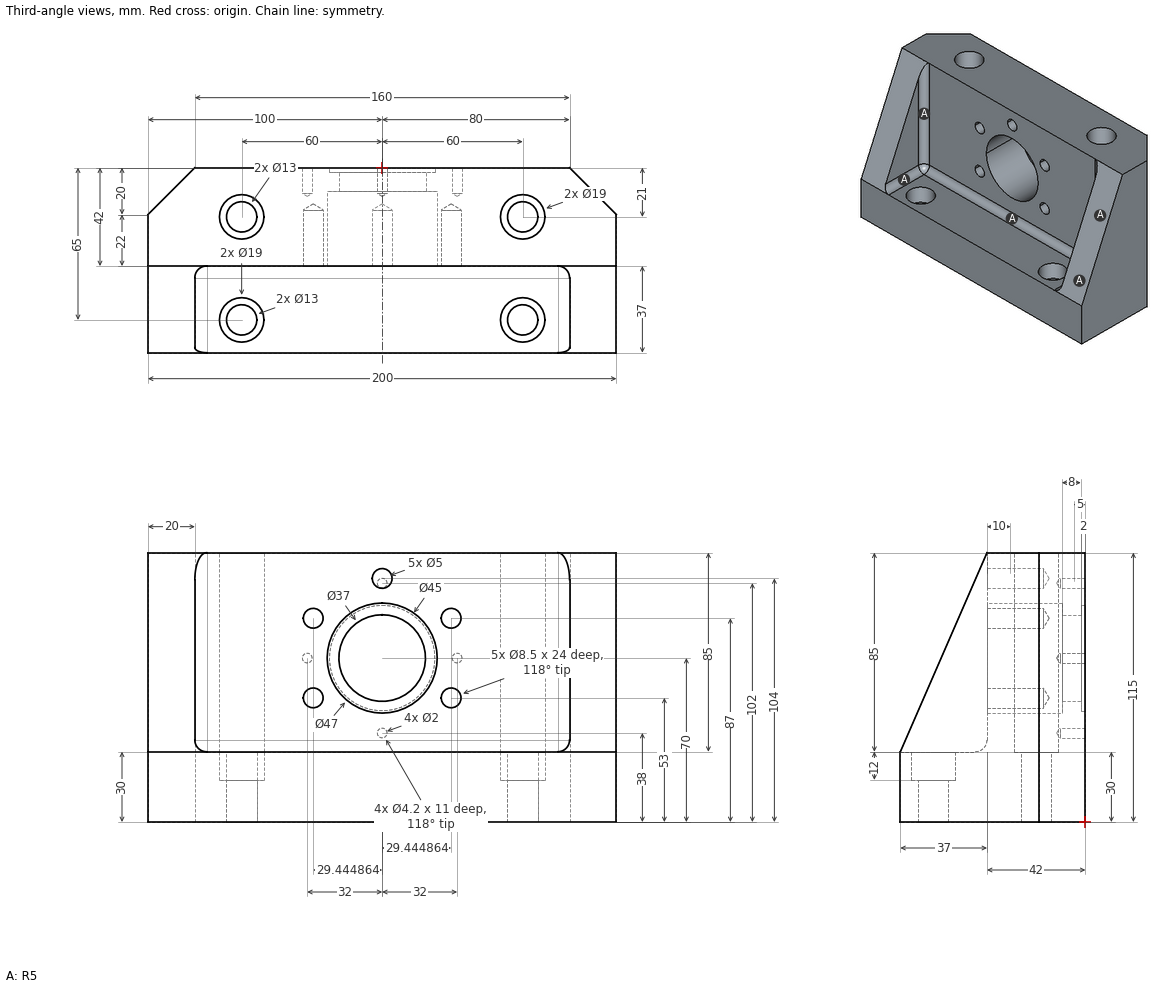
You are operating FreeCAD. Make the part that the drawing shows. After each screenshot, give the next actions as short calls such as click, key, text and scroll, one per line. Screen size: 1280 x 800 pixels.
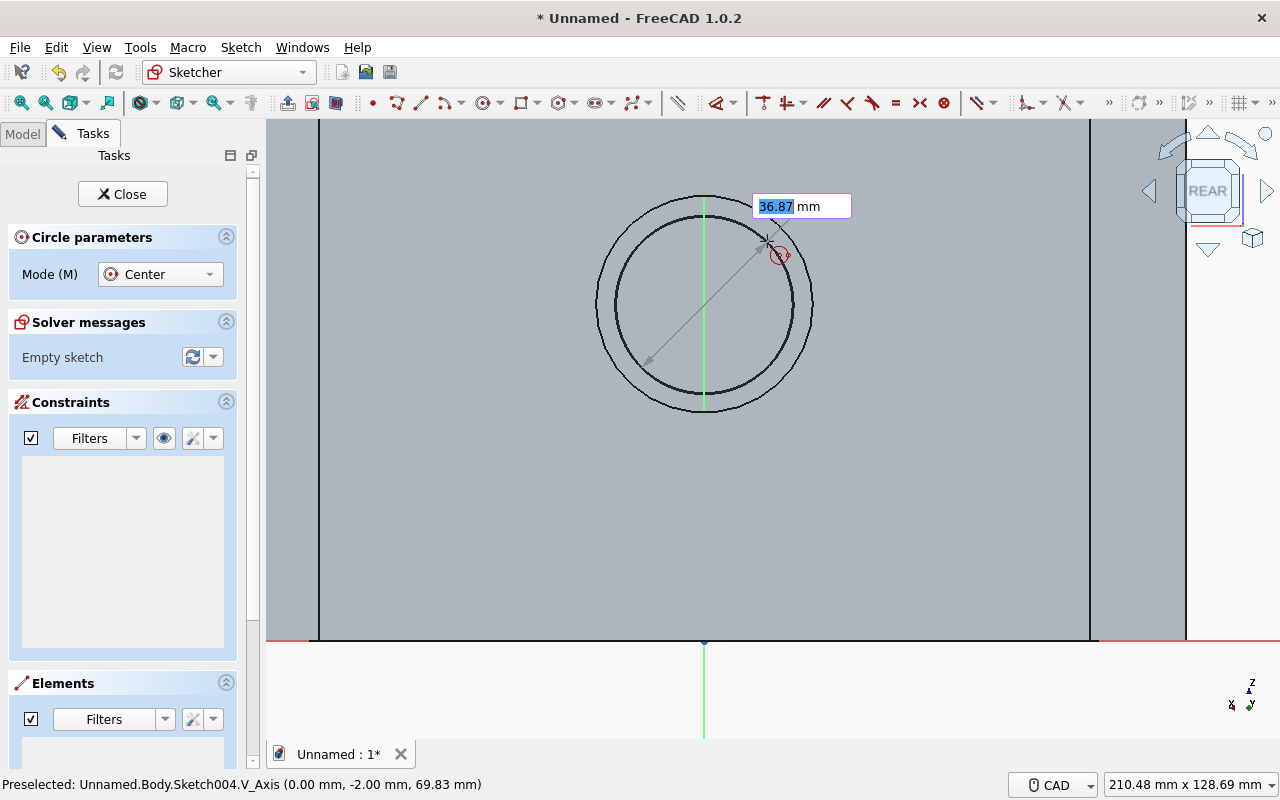
text(37)
key(Return)
key(Escape)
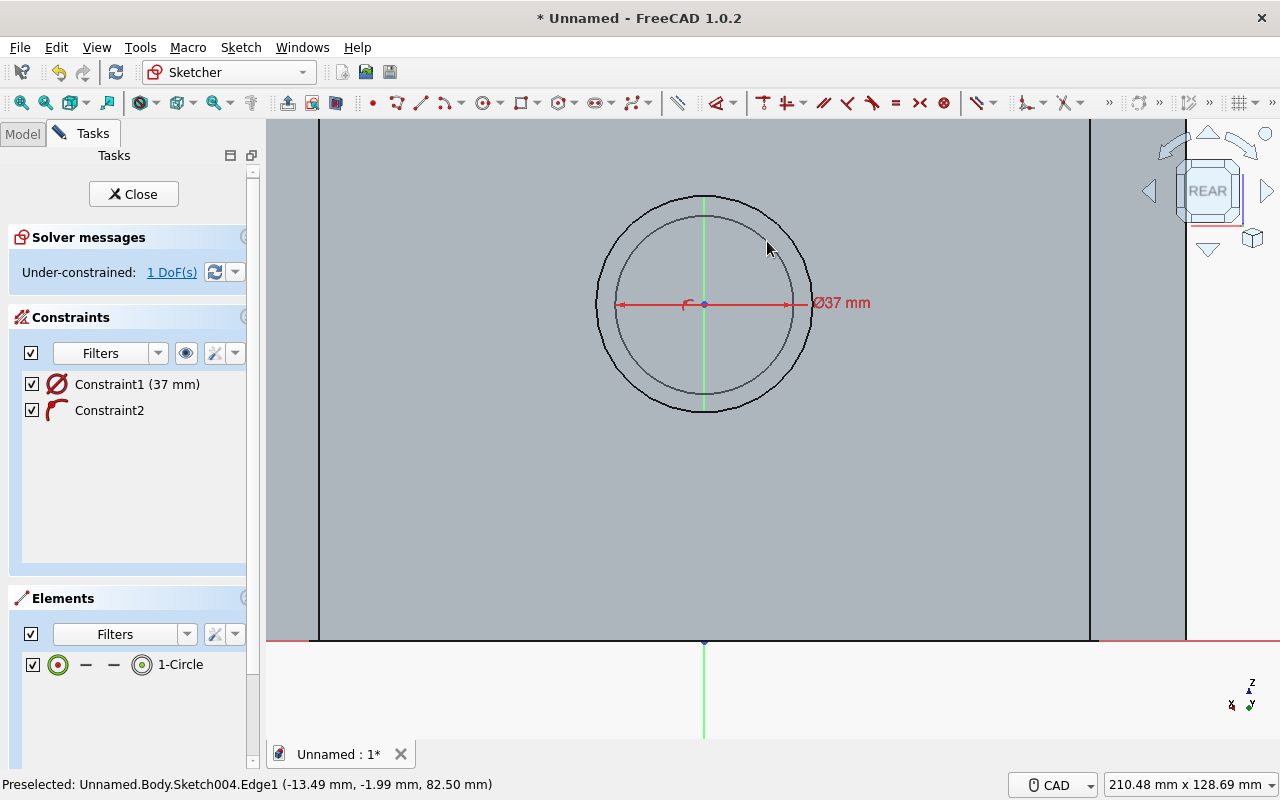
click(716, 104)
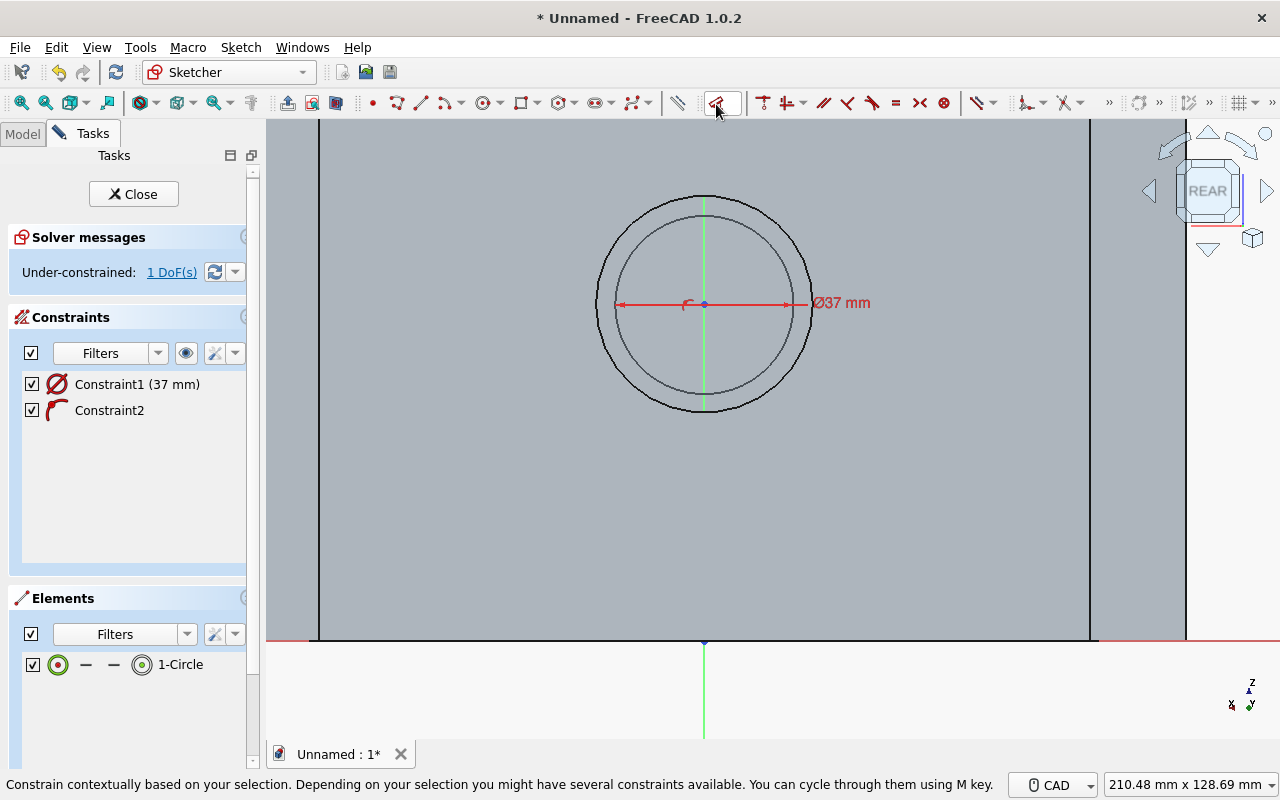
click(704, 305)
click(738, 473)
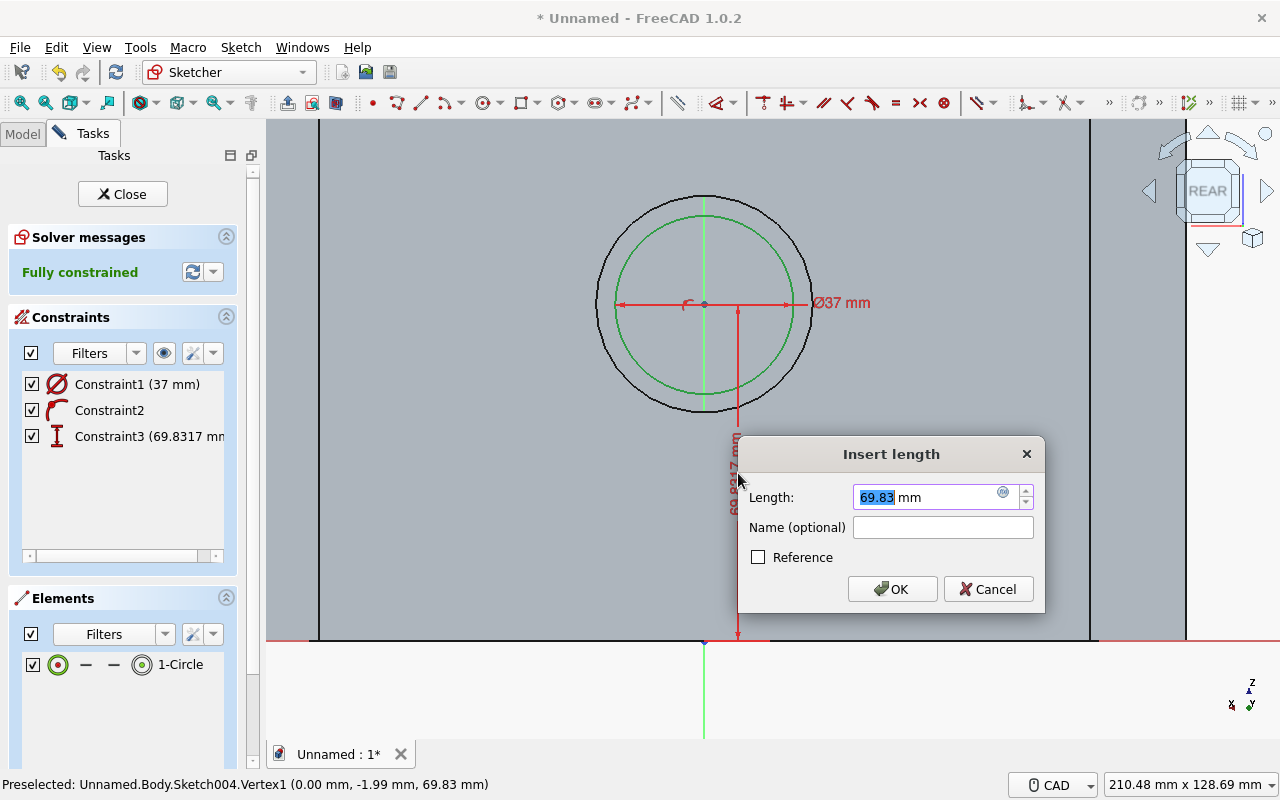
text(70)
key(Return)
key(Escape)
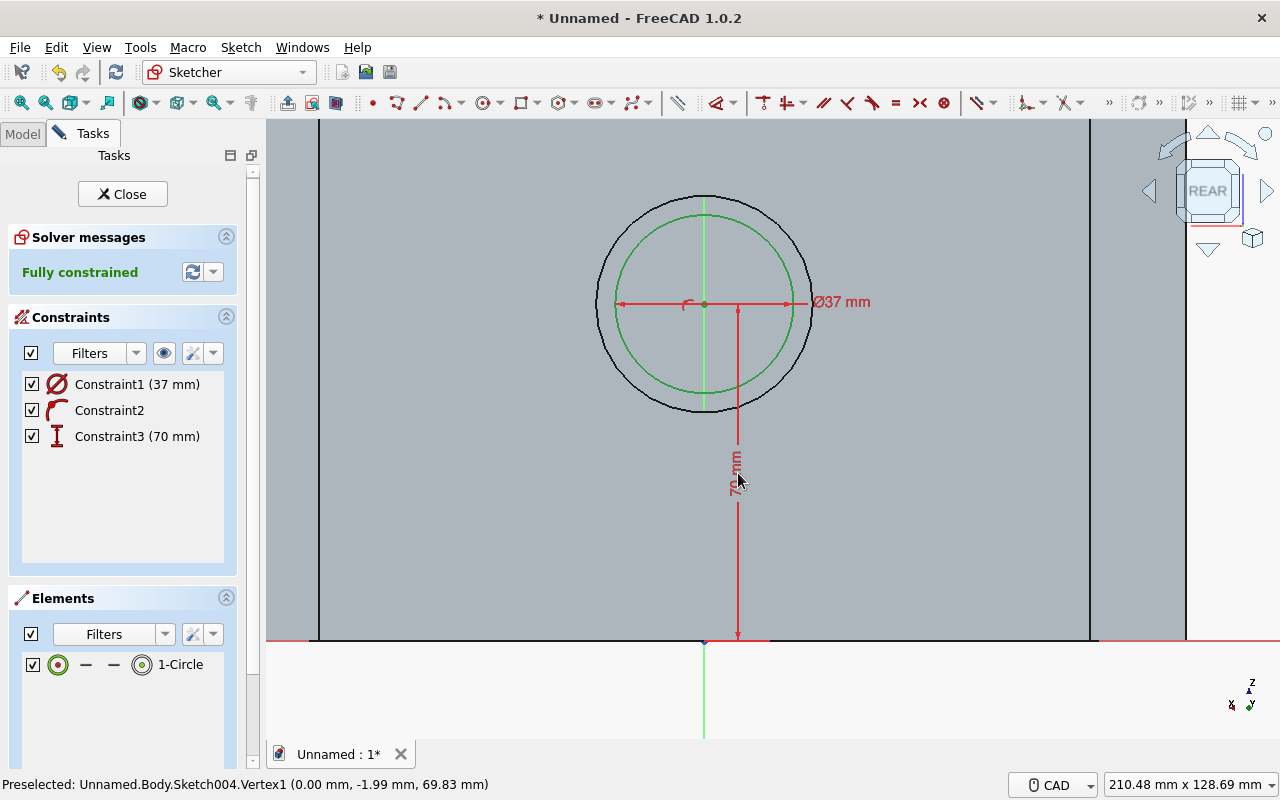
click(123, 194)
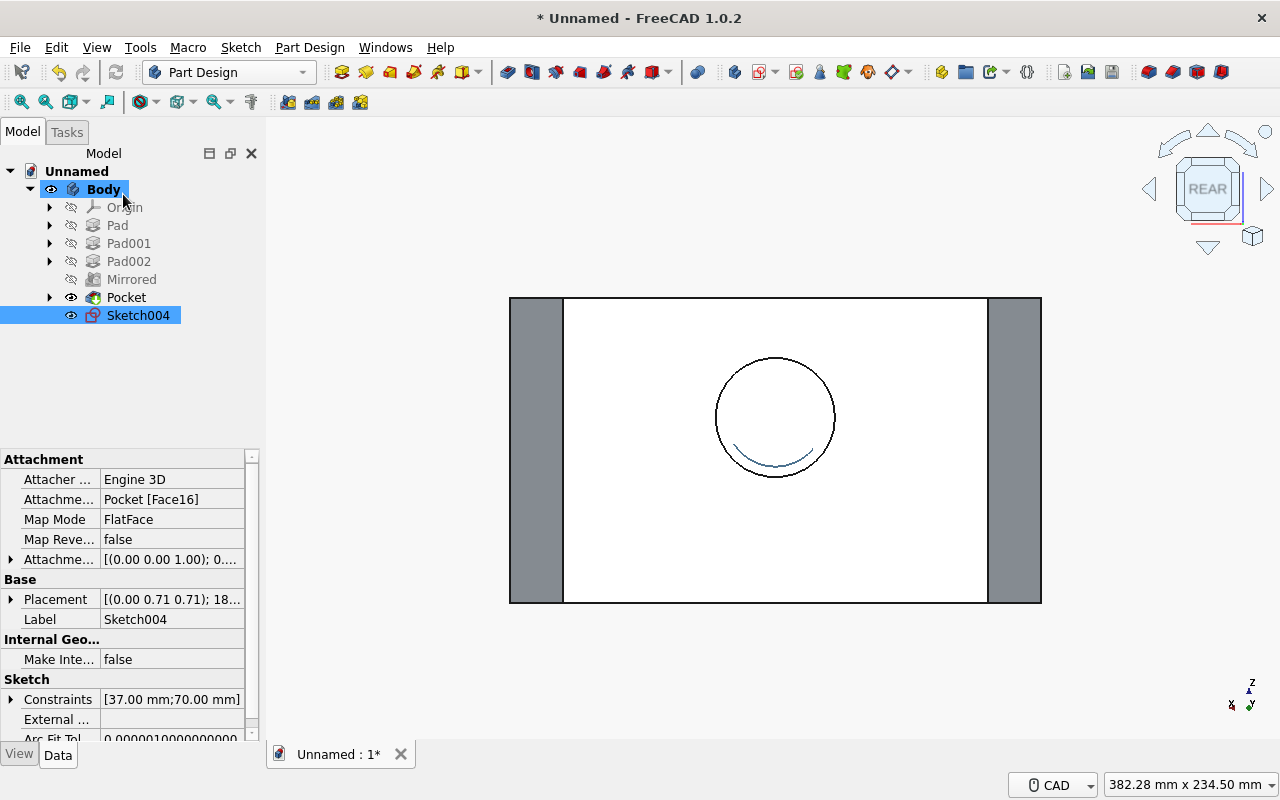
click(508, 72)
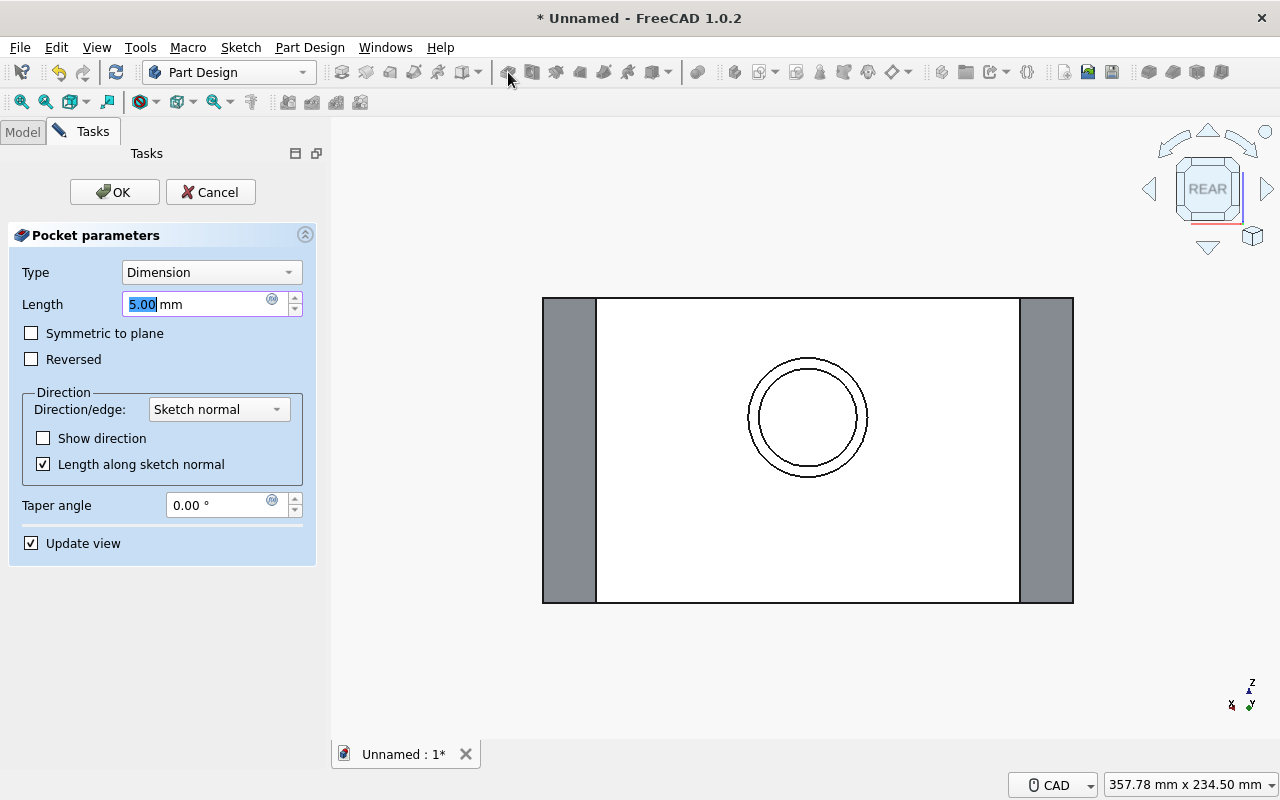
text(8)
key(Tab)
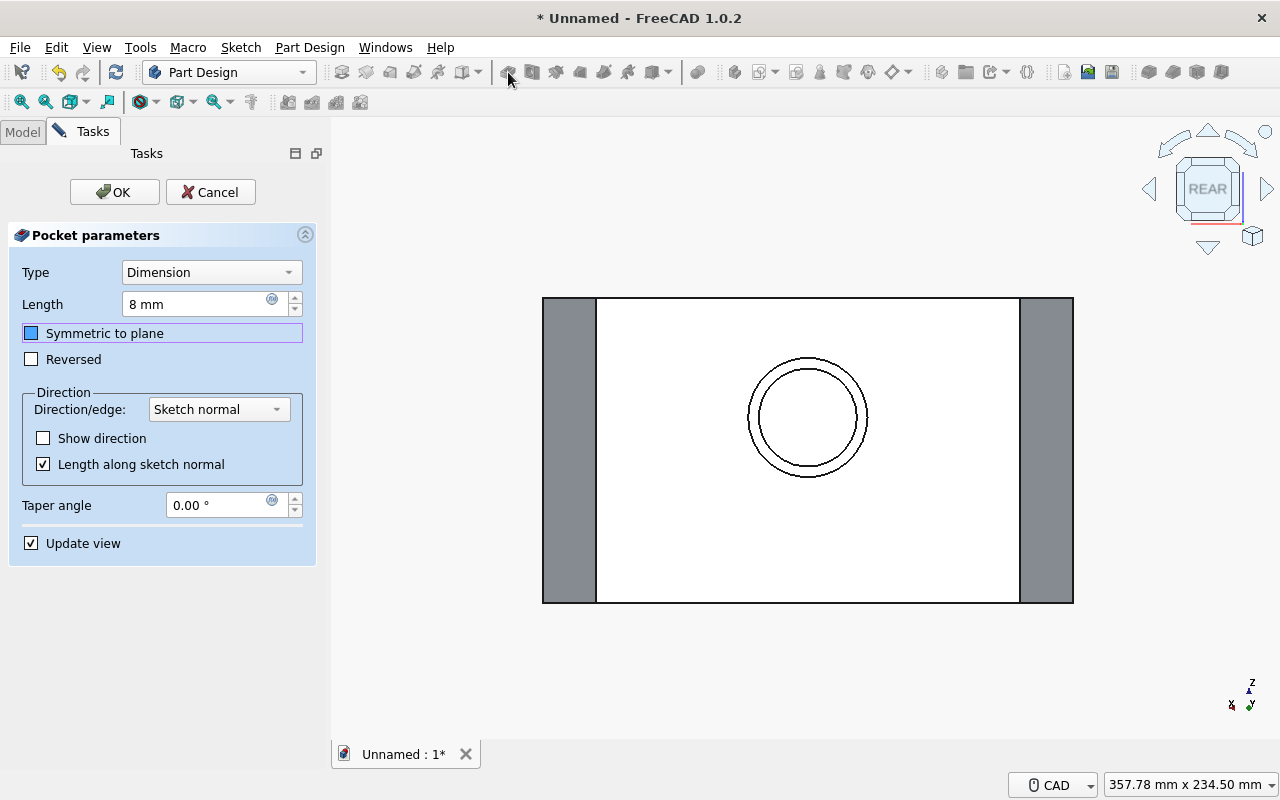
click(115, 192)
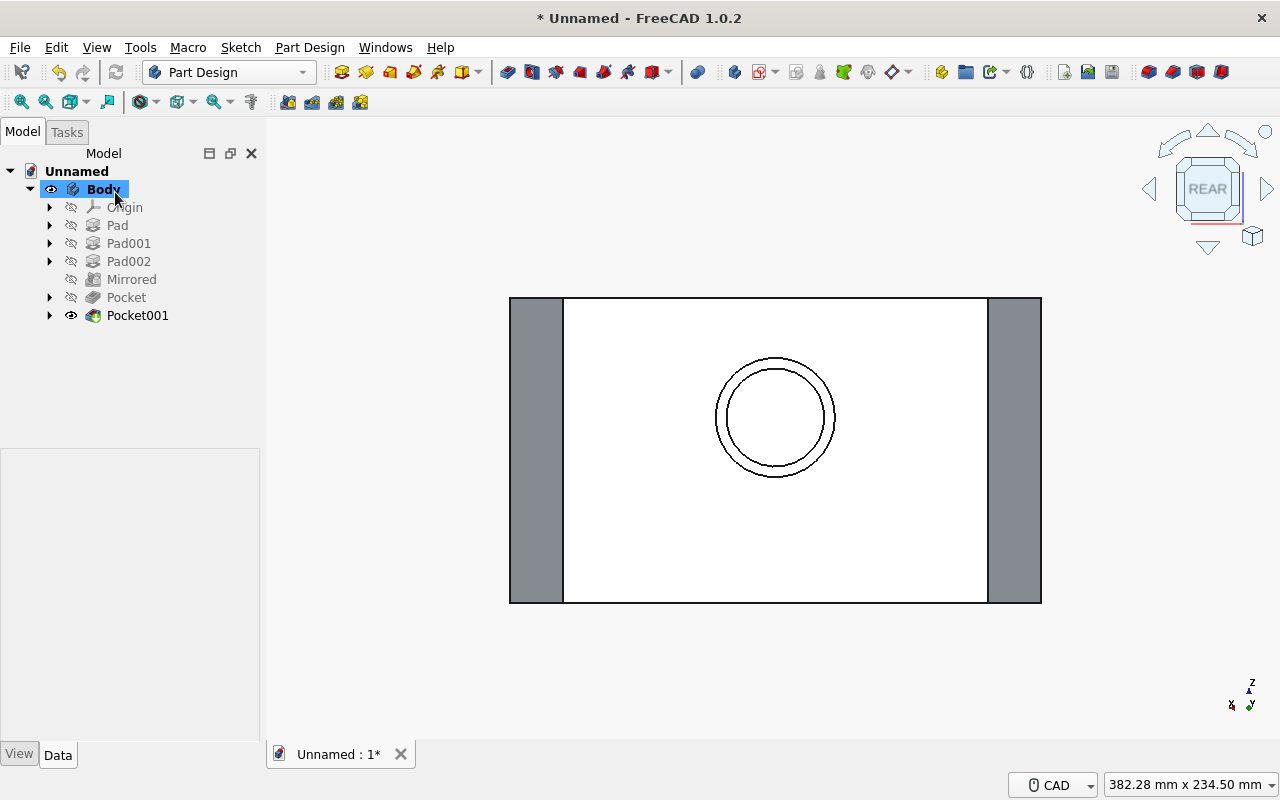
click(775, 417)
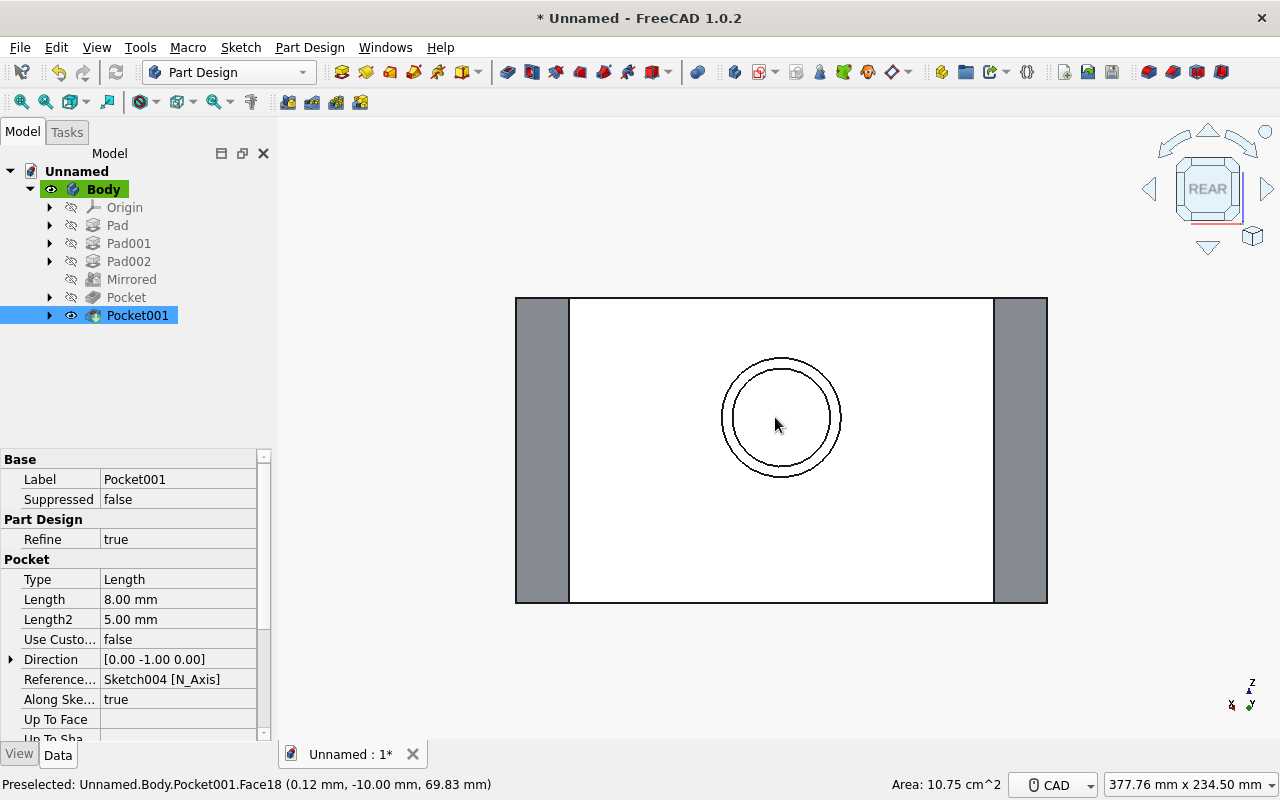
click(760, 72)